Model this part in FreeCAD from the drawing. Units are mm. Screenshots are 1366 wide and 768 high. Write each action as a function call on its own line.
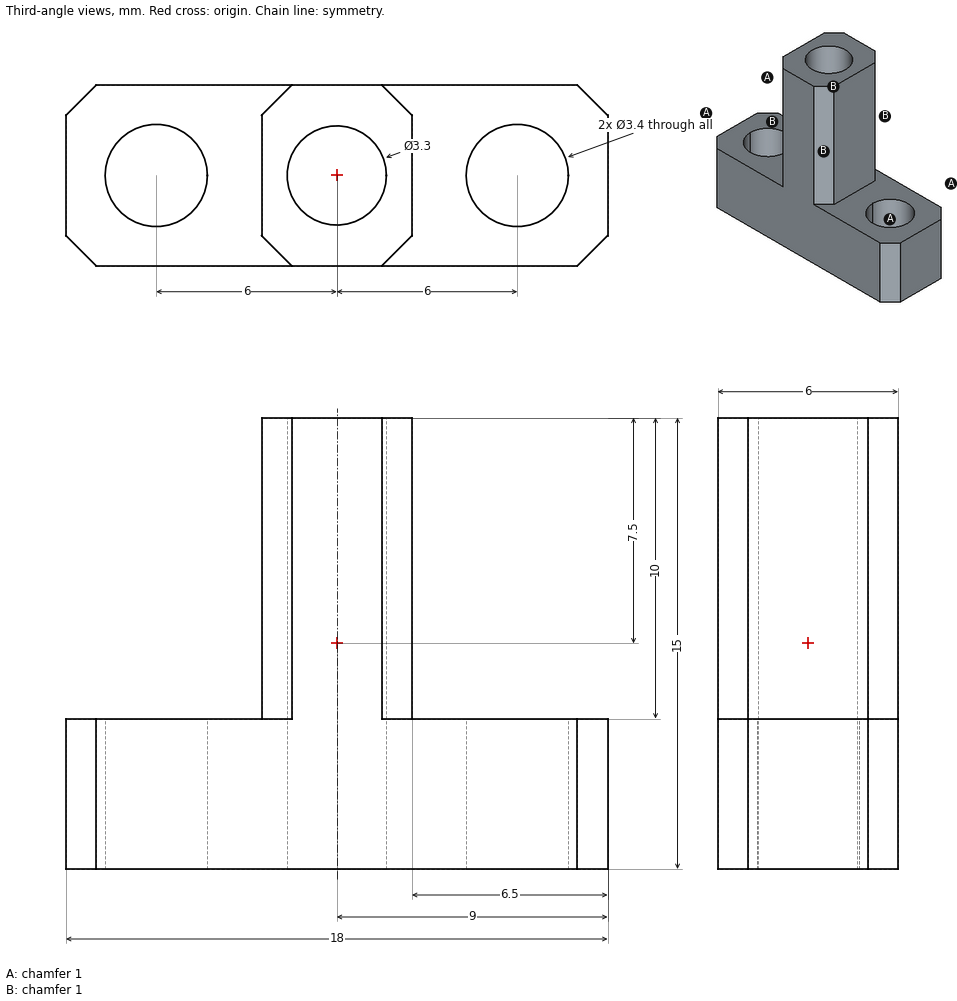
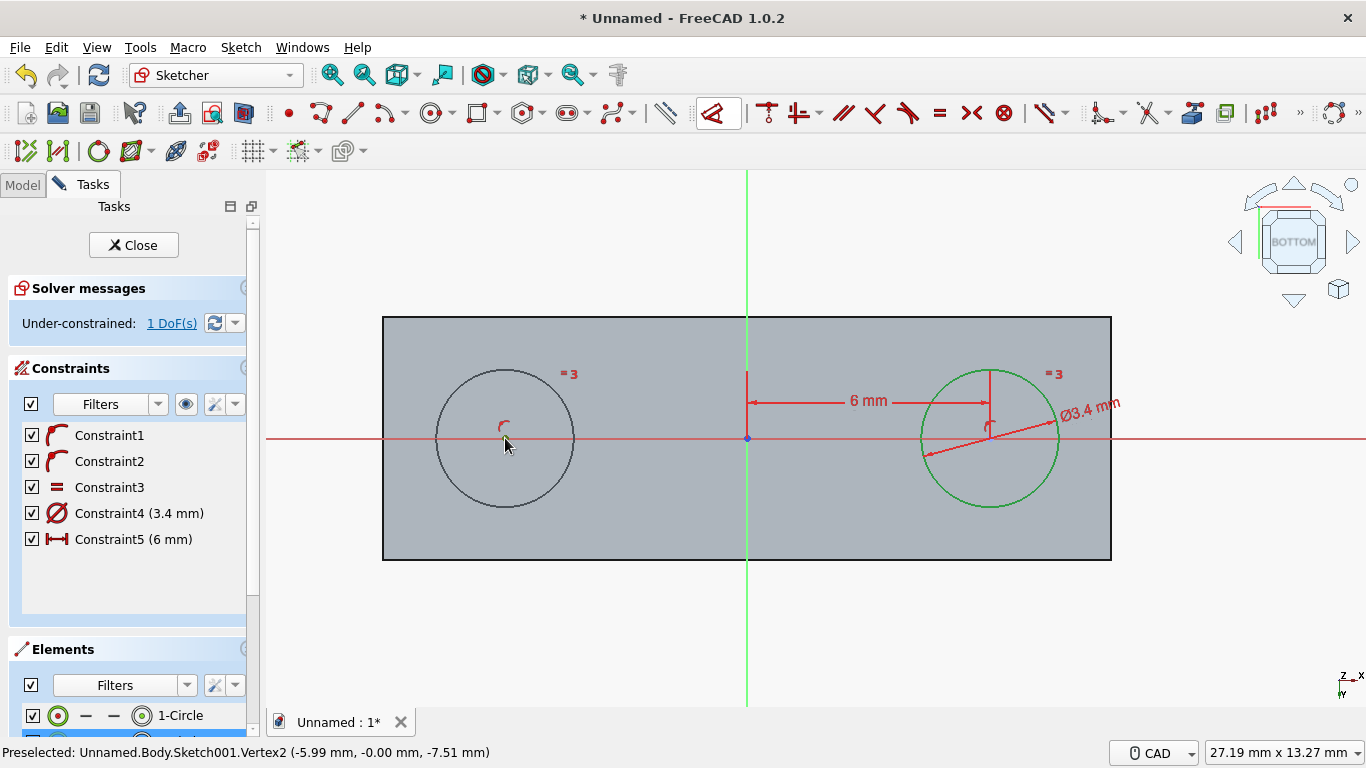
key(l)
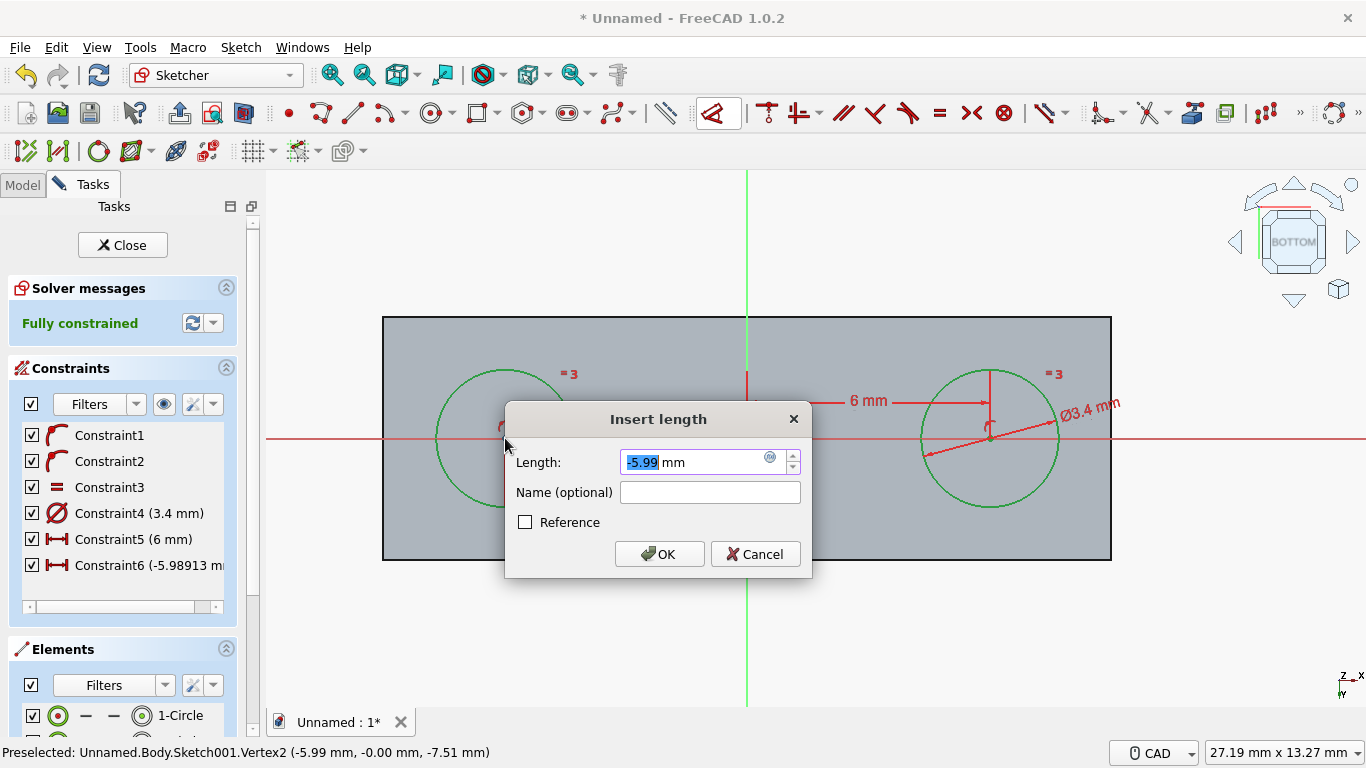
text(-6)
key(Return)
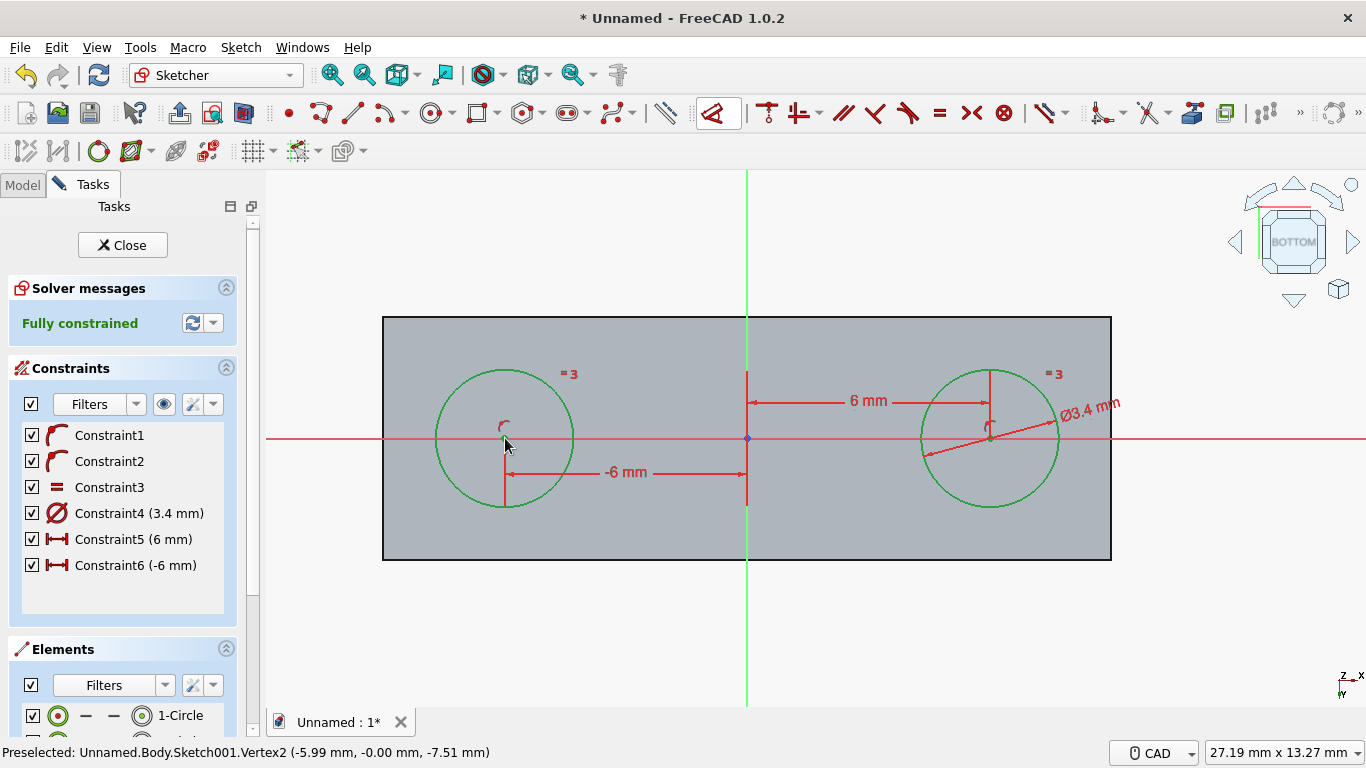
click(123, 245)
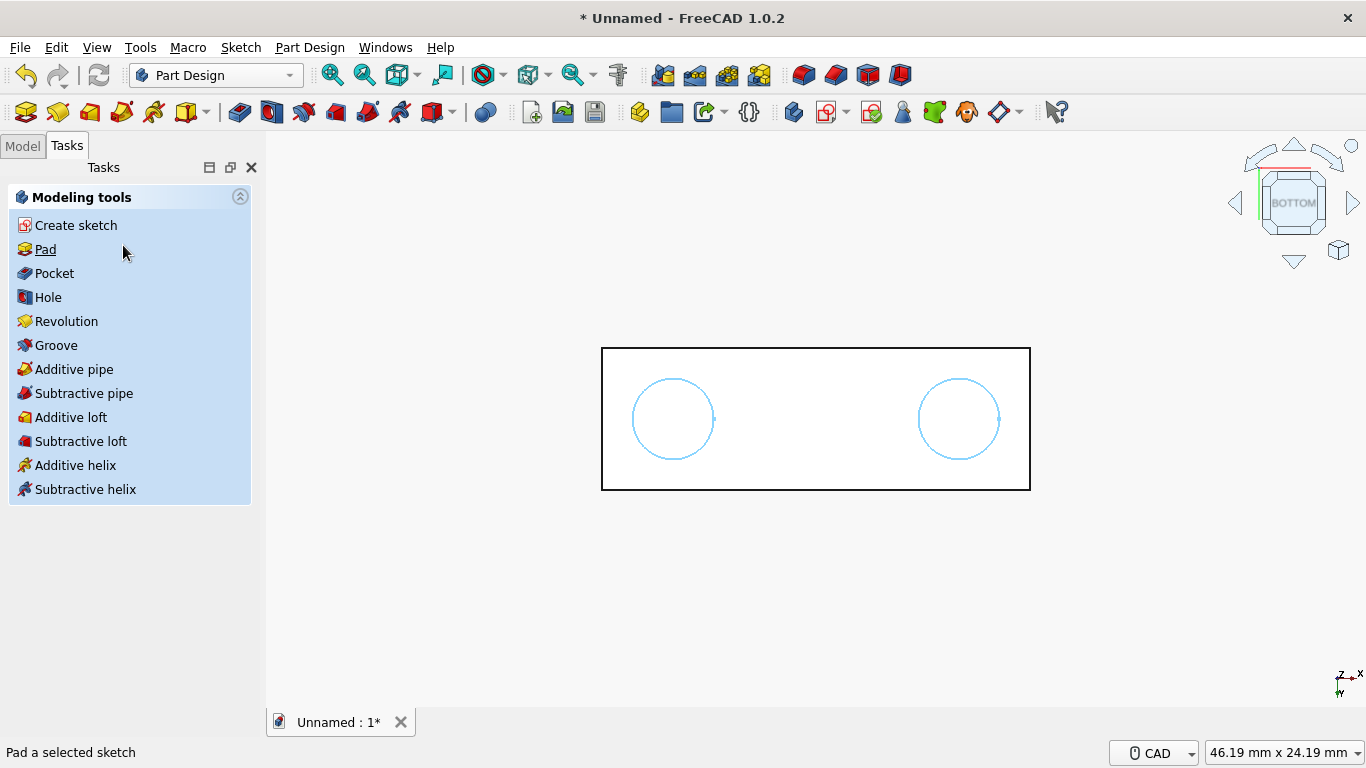
click(272, 112)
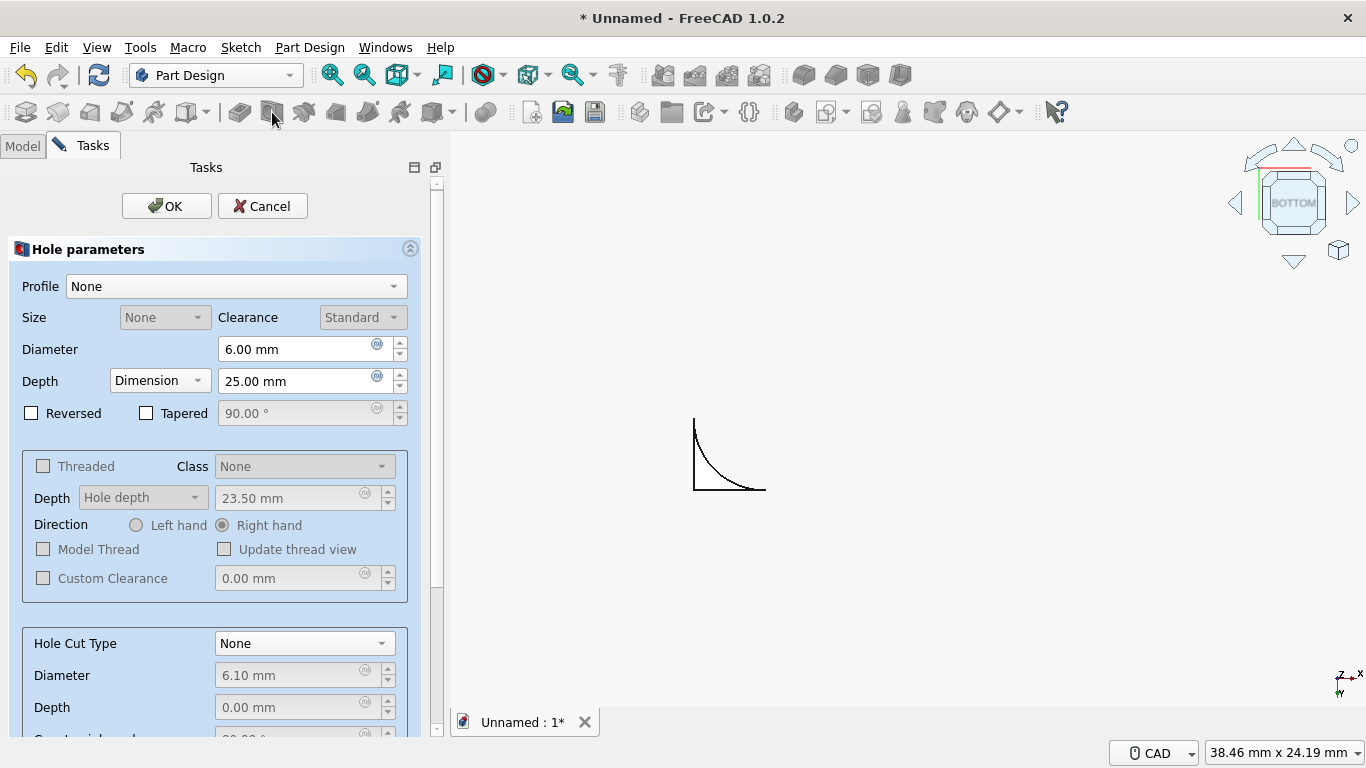
triple_click(305, 349)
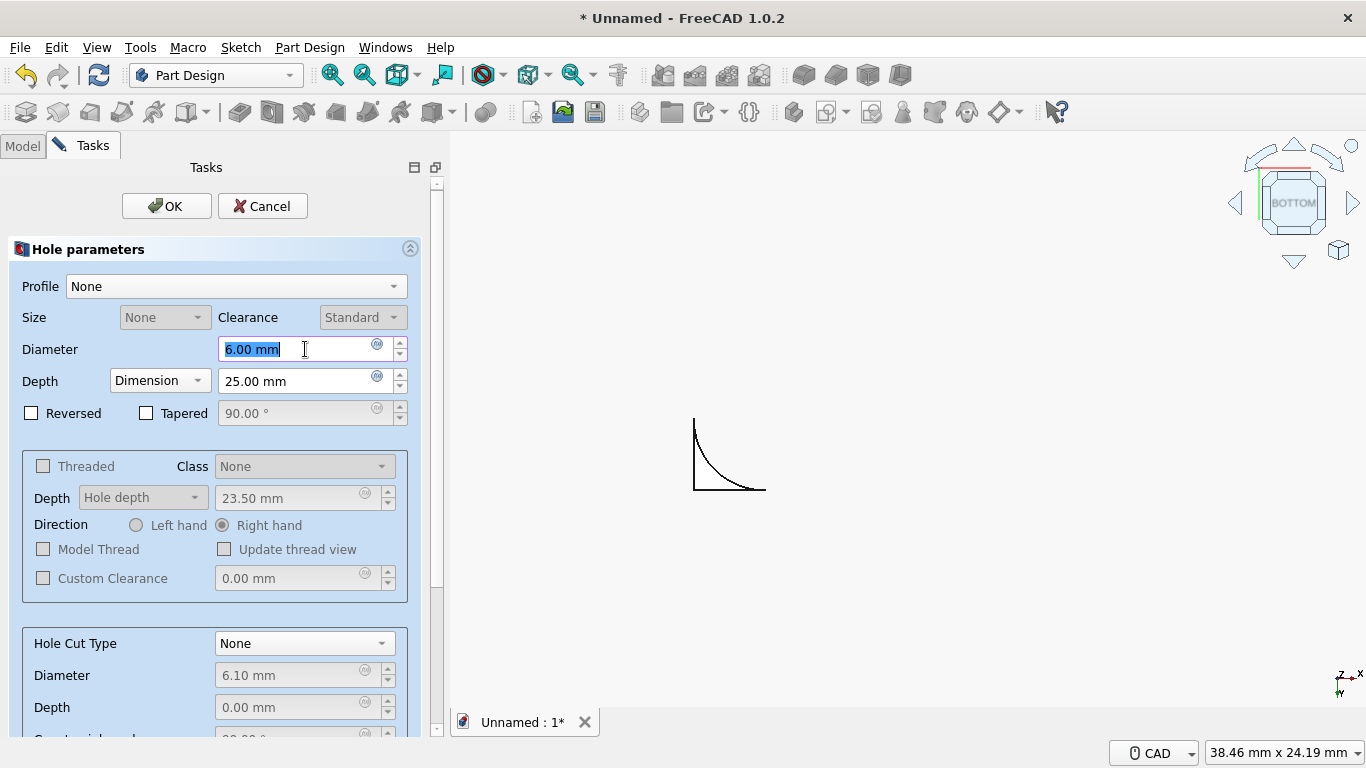
text(3.4)
key(Tab)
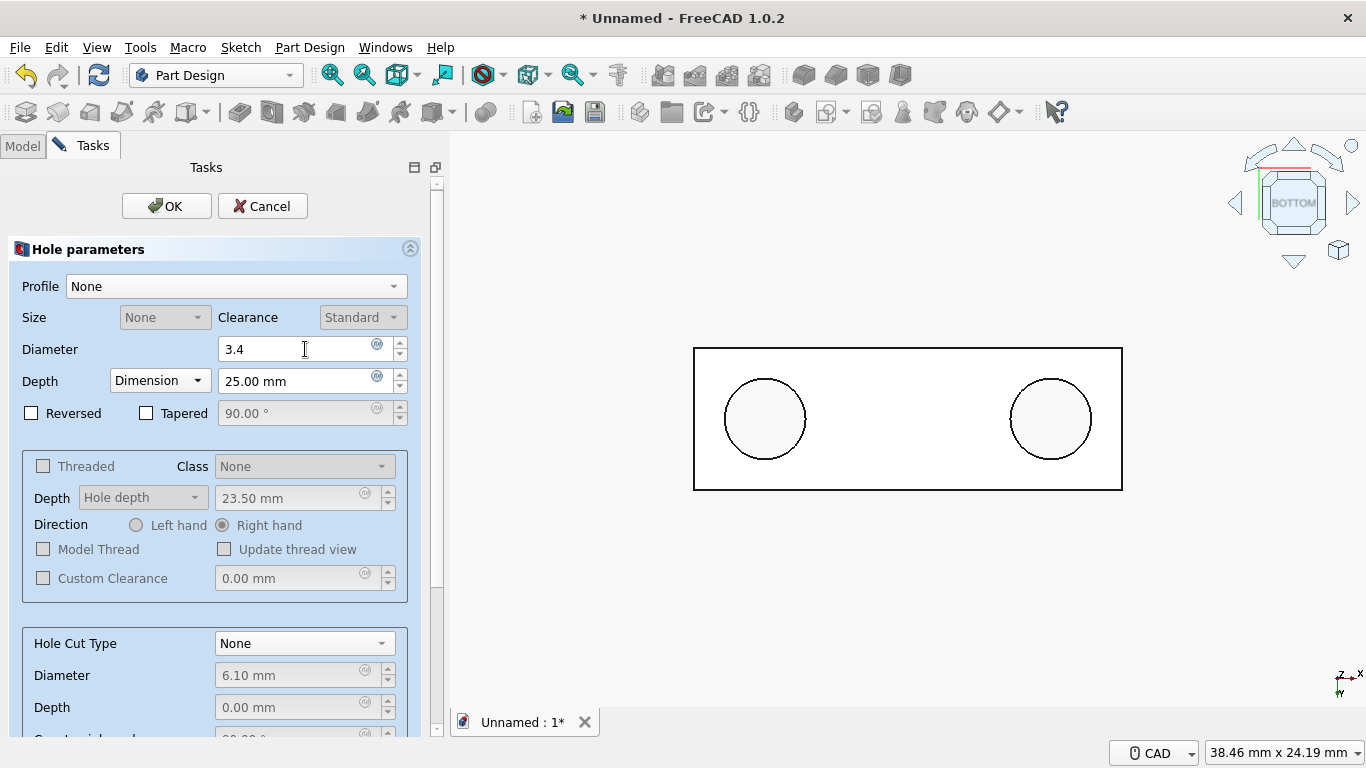
click(161, 380)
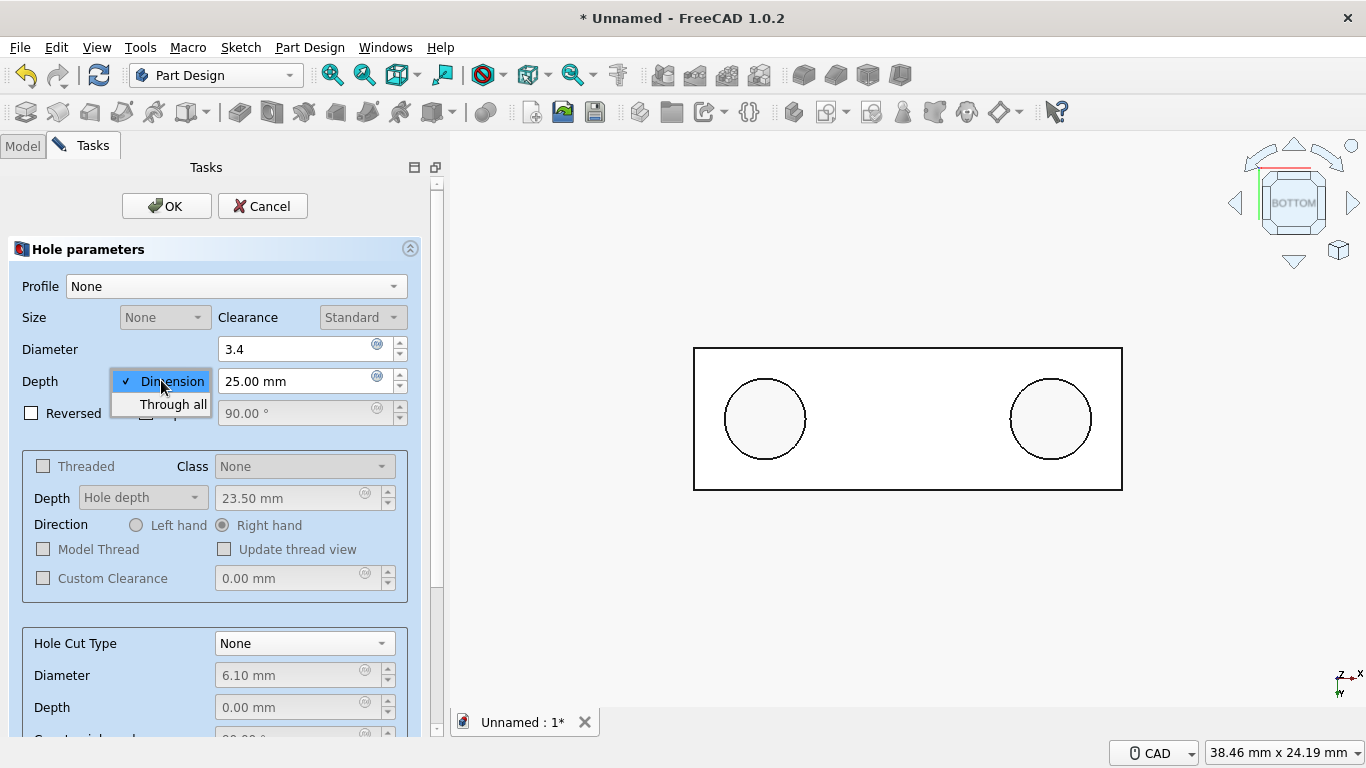
click(160, 404)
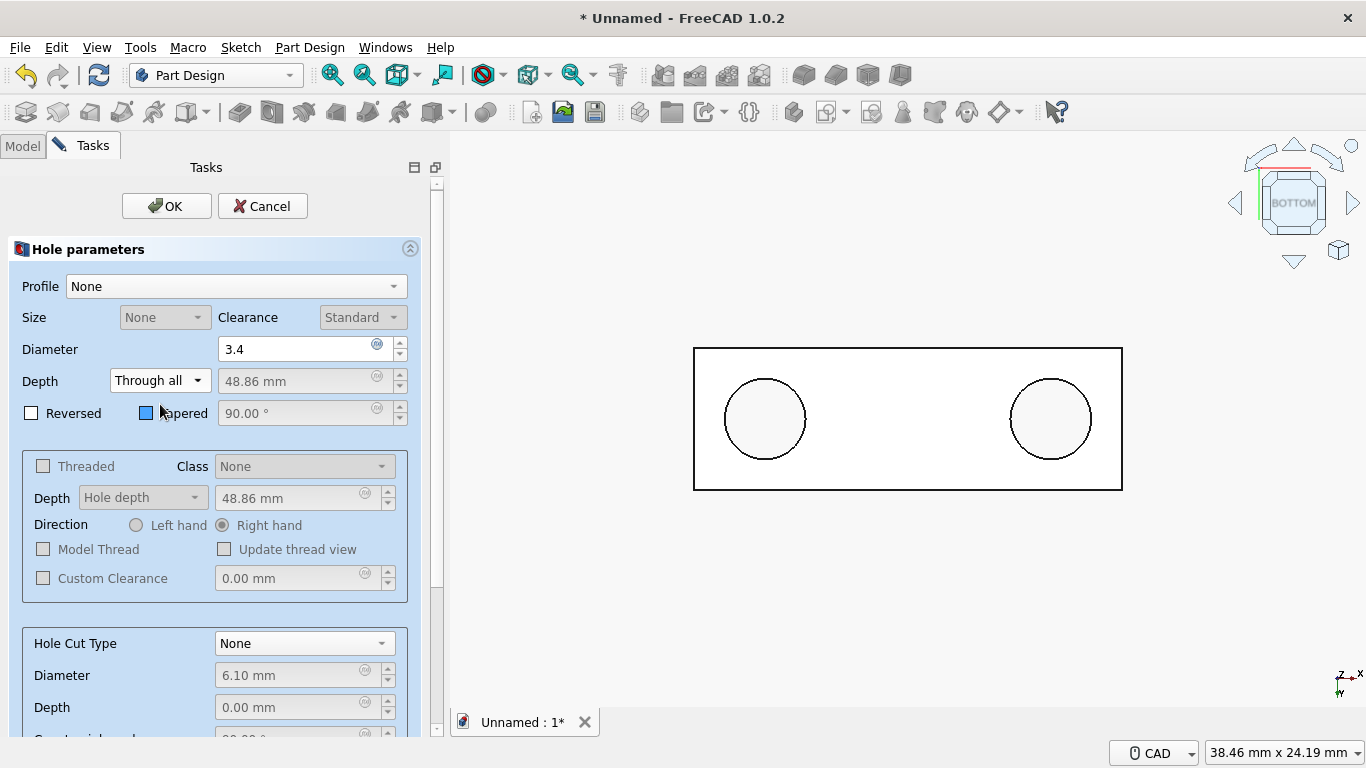
click(167, 206)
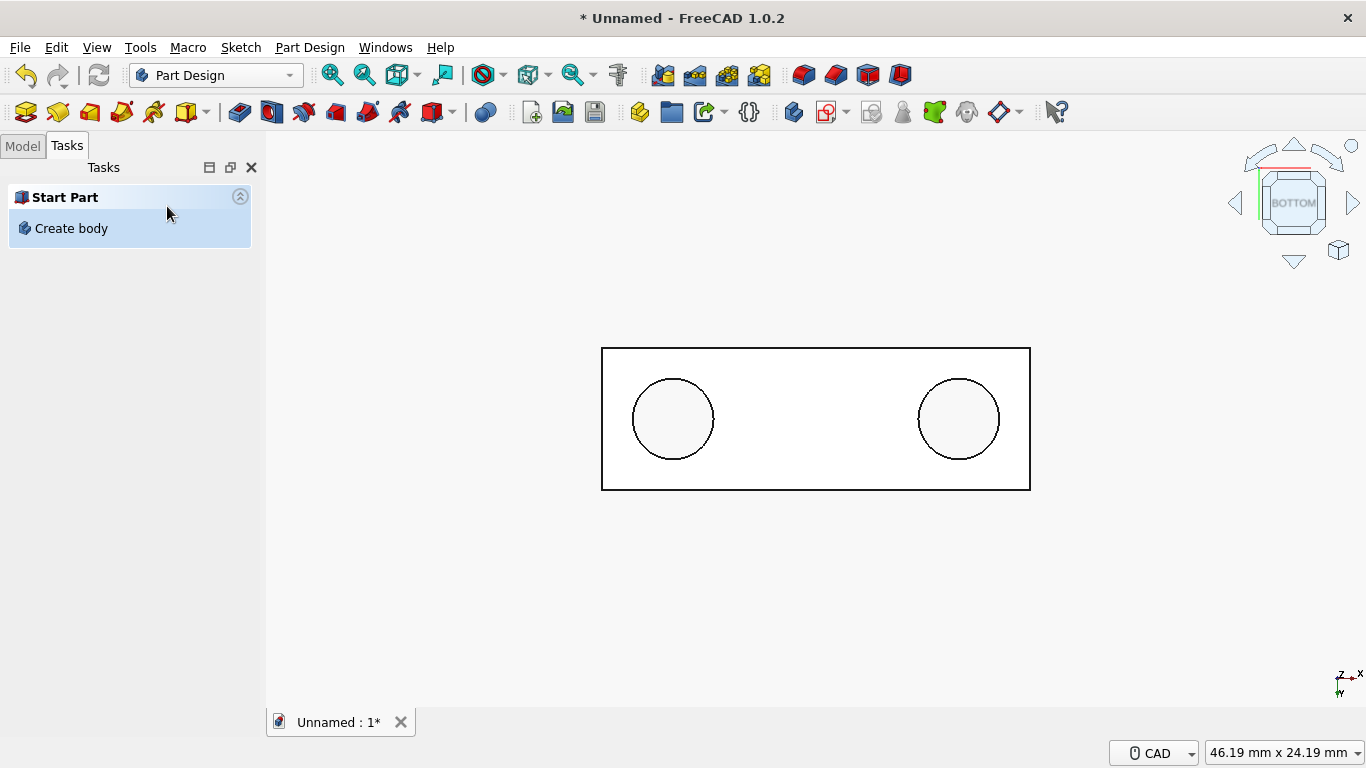
click(334, 76)